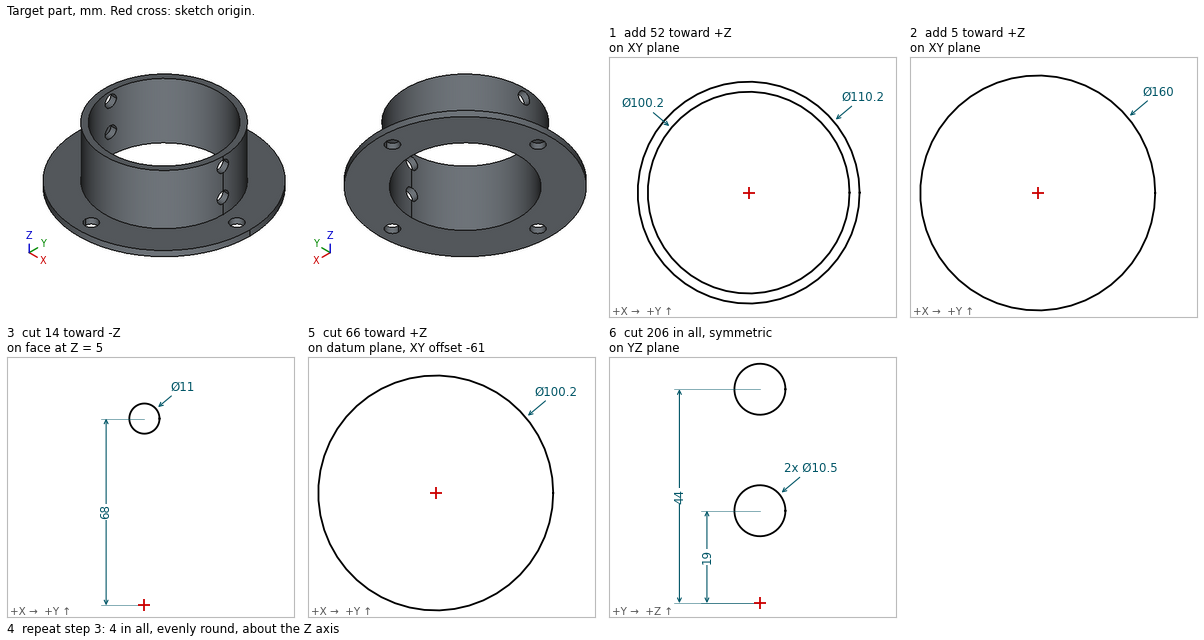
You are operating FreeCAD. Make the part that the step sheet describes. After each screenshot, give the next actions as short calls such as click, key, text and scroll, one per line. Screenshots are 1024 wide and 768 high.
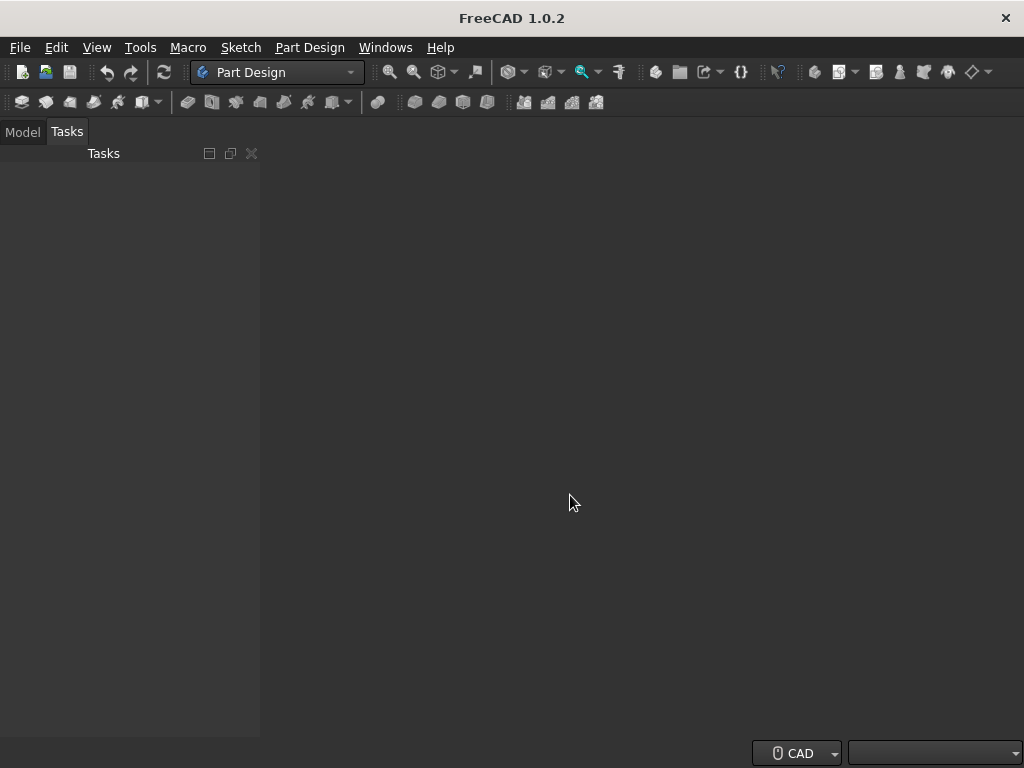
click(22, 72)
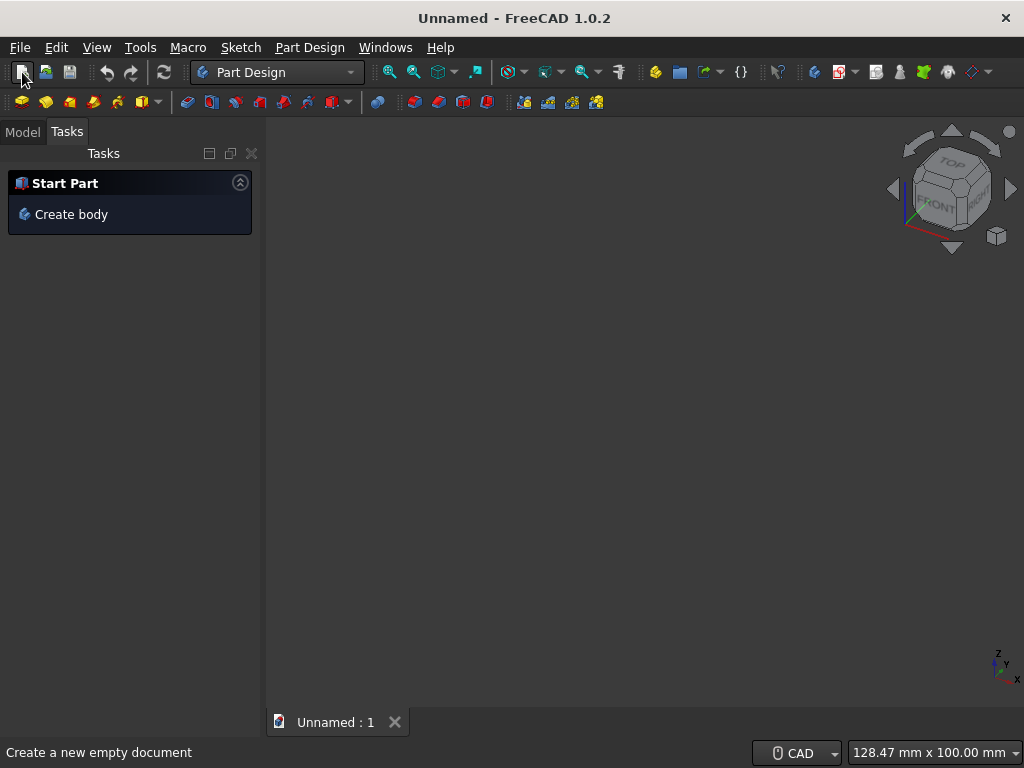
click(840, 72)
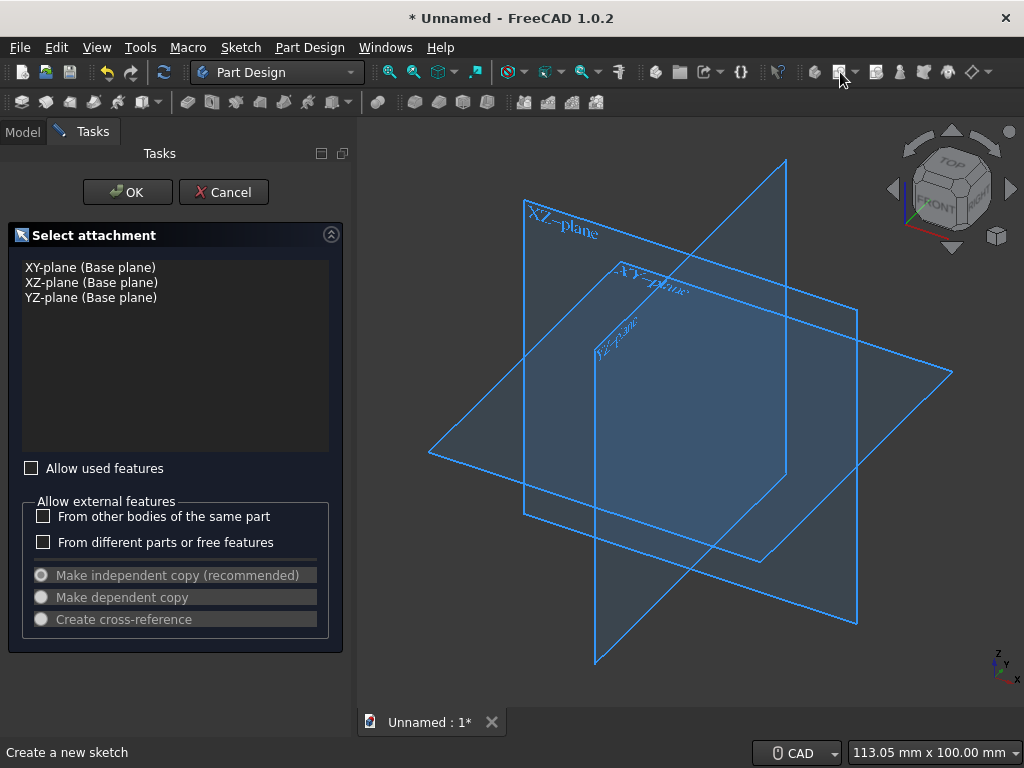
click(82, 268)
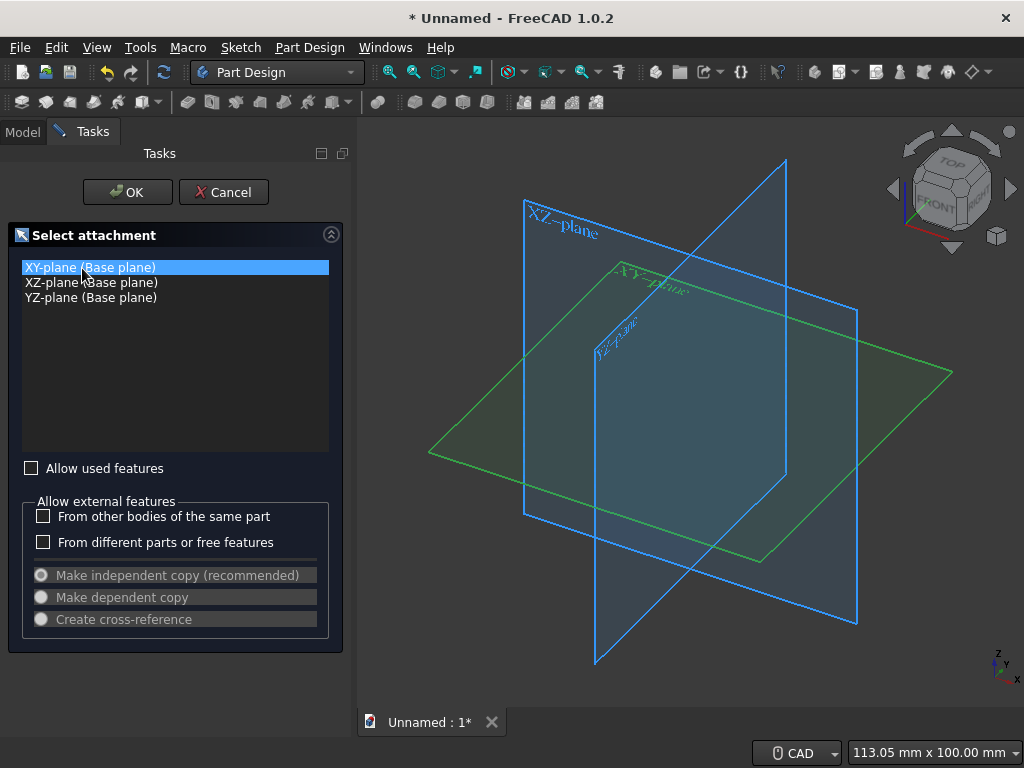
click(128, 192)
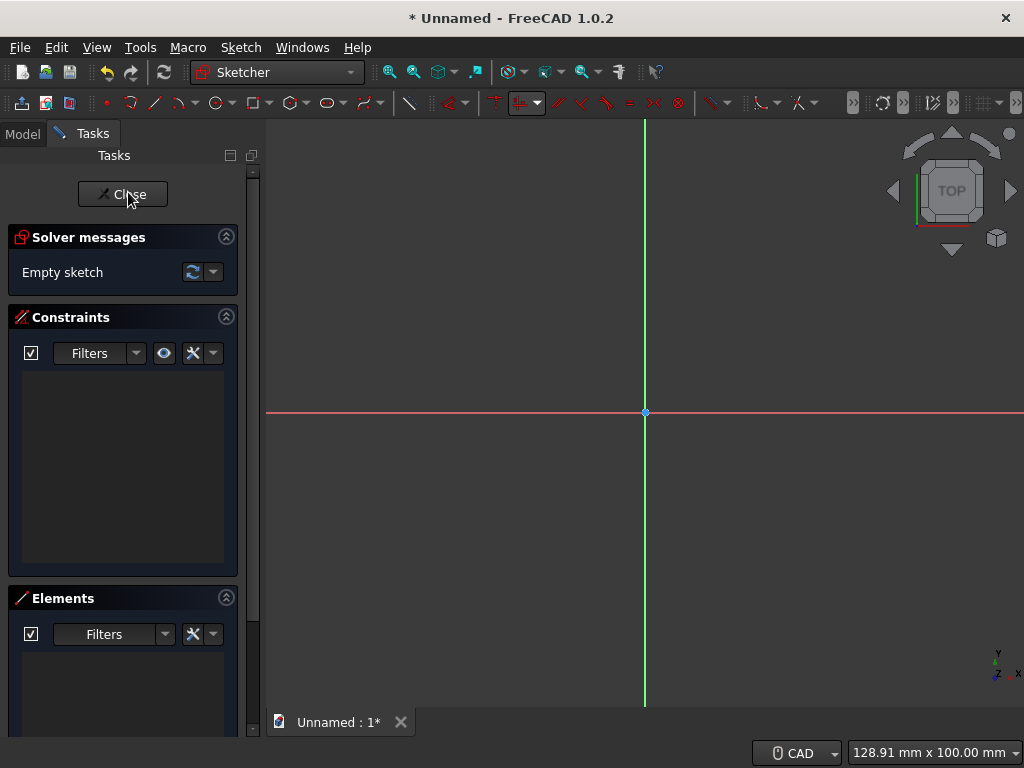
scroll(493, 413, down, 3)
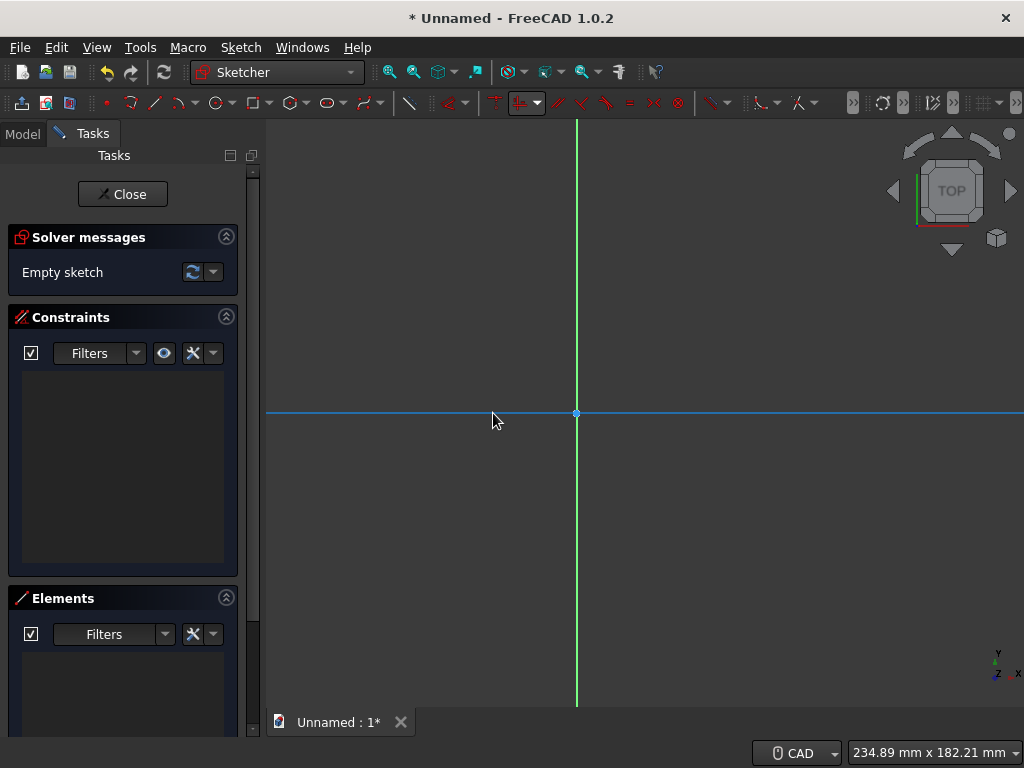
click(216, 104)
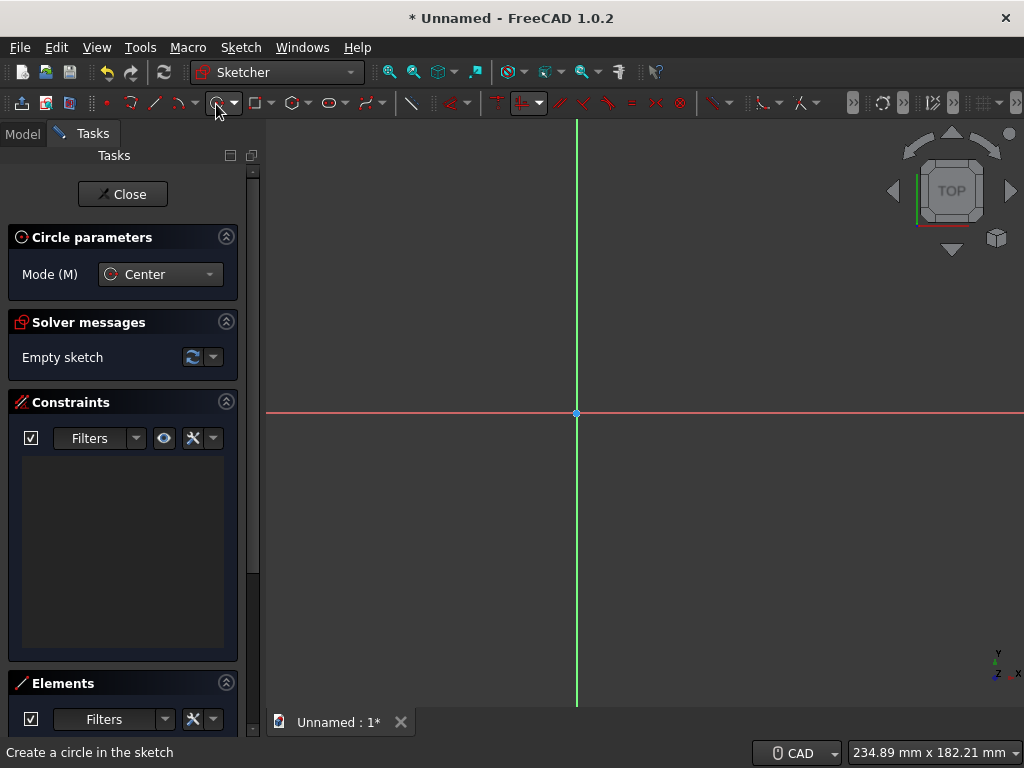
click(577, 413)
click(702, 287)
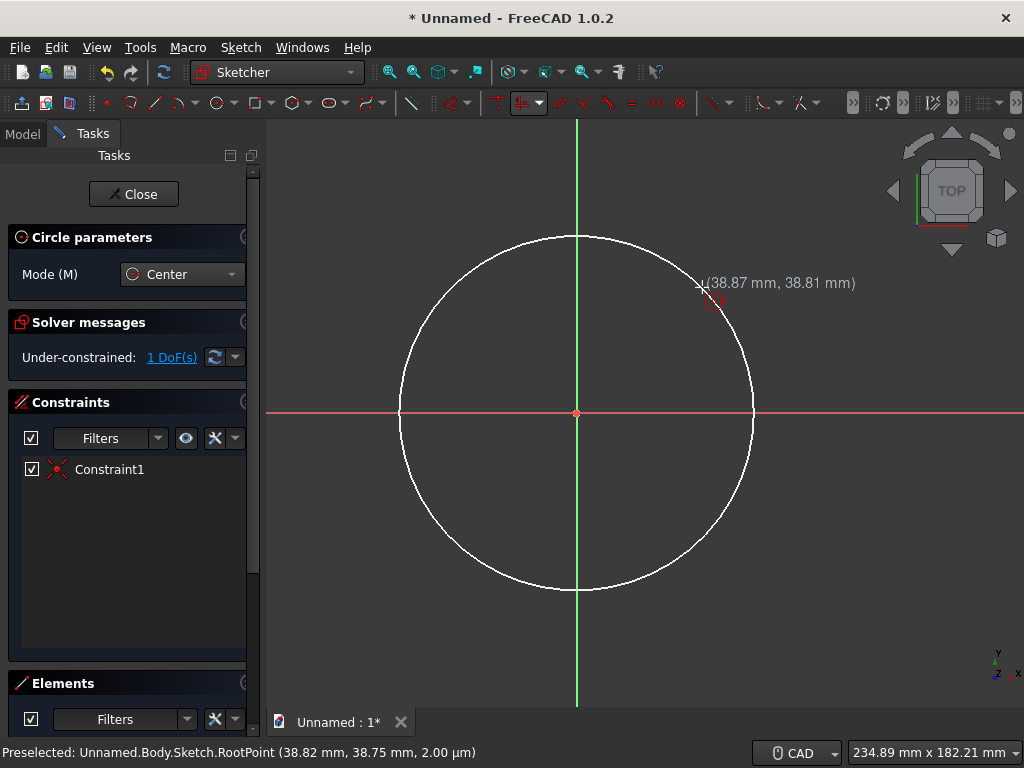
click(577, 413)
click(691, 299)
key(Escape)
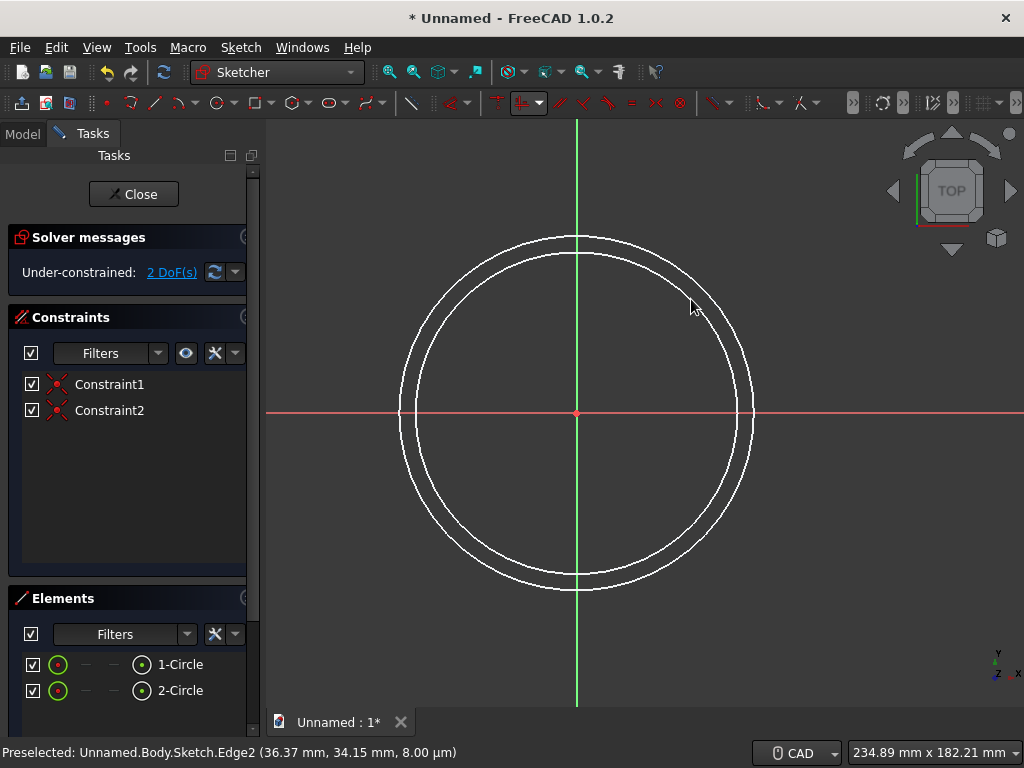
click(450, 104)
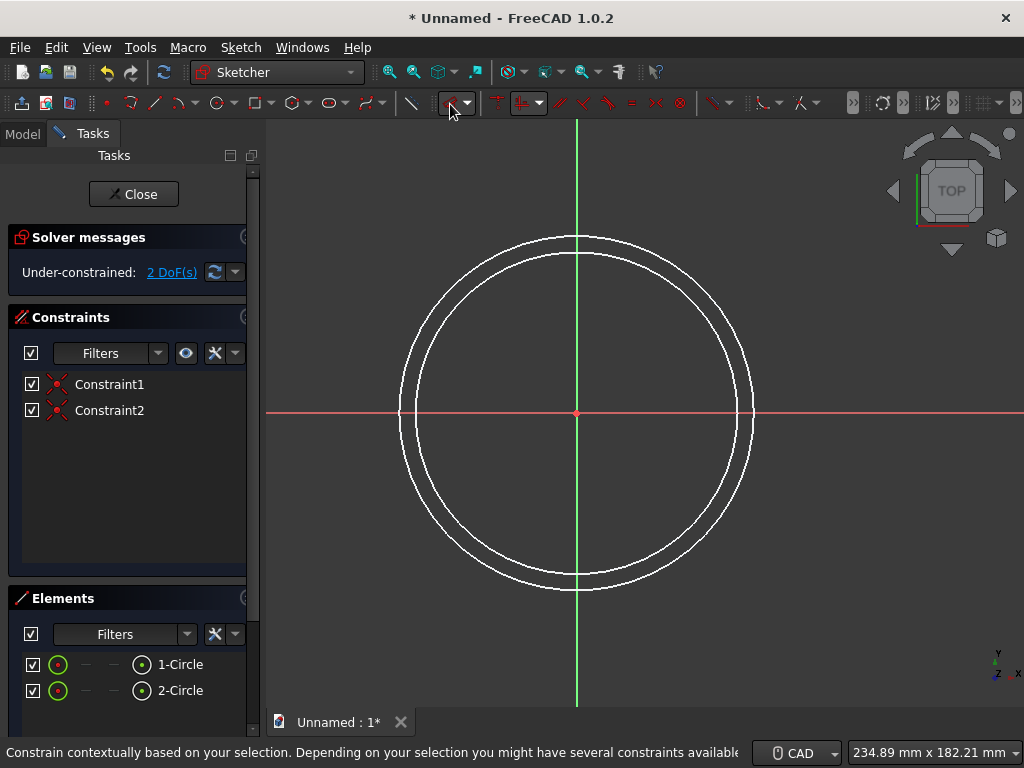
click(702, 288)
click(725, 265)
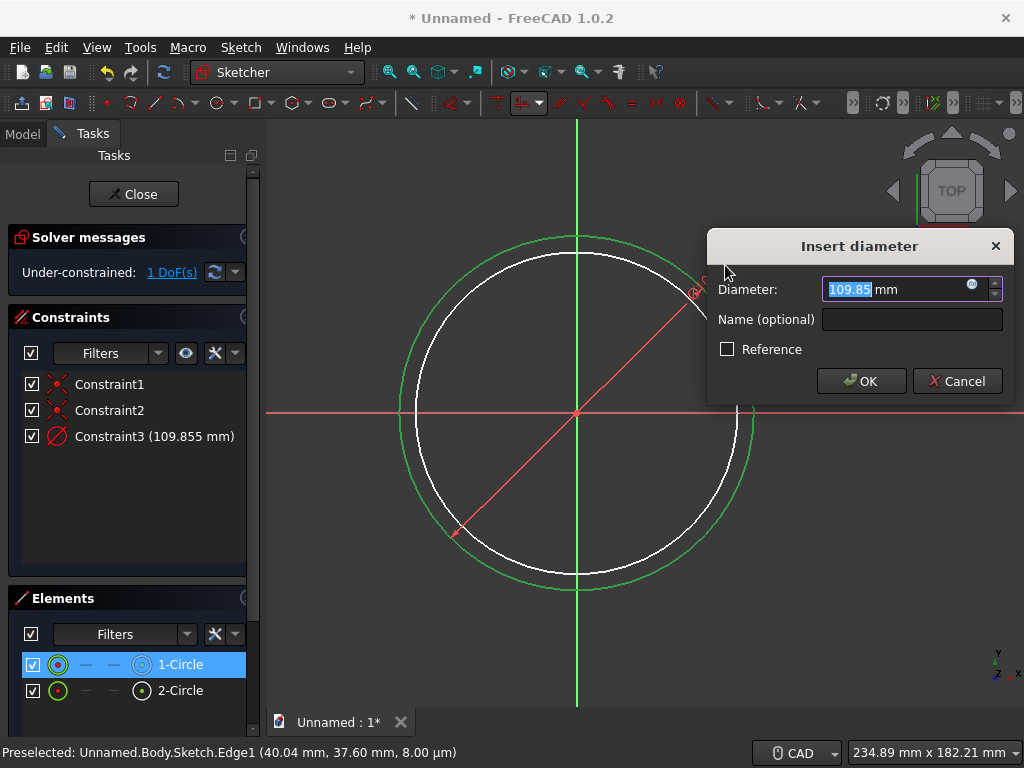
text(110.2)
key(Return)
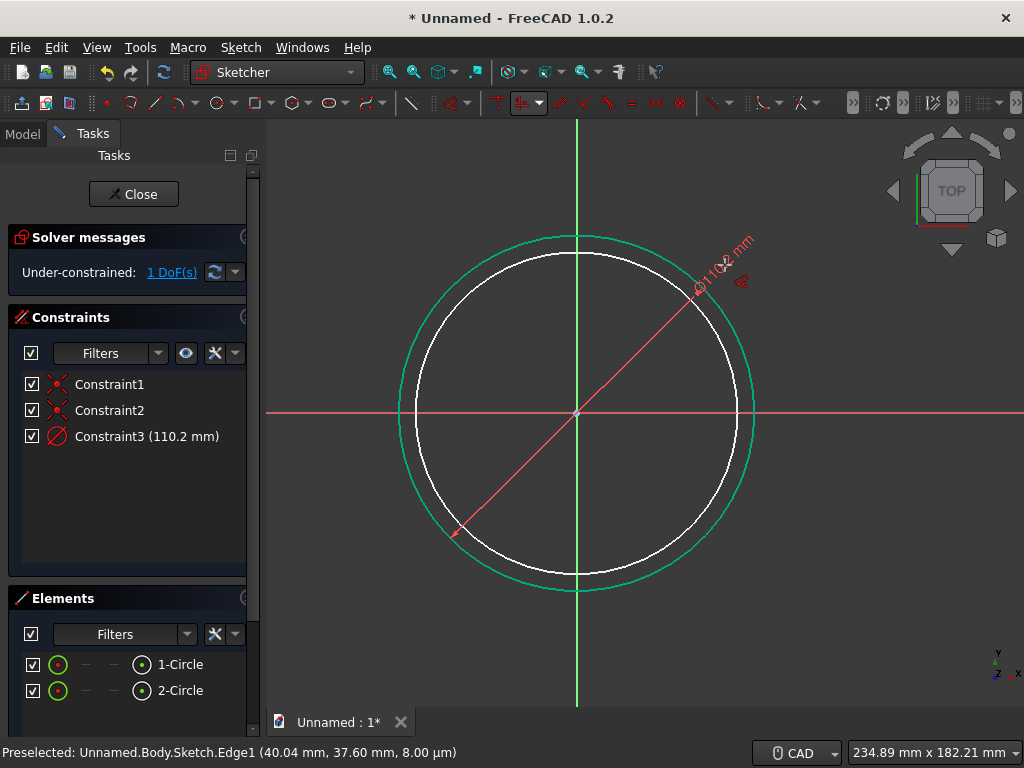
click(690, 299)
click(762, 358)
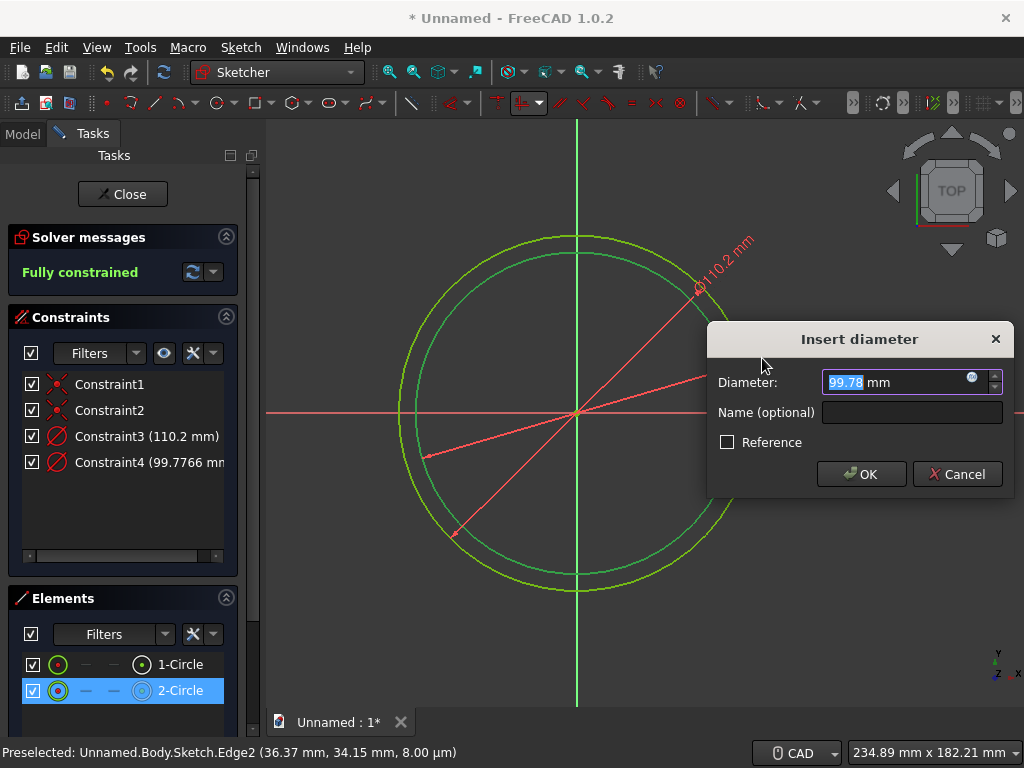
text(100.2)
key(Return)
key(Escape)